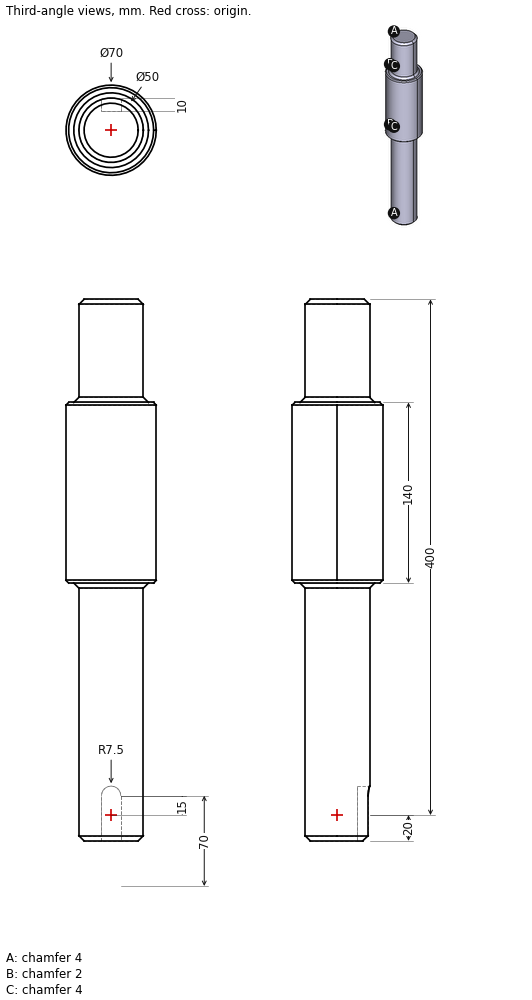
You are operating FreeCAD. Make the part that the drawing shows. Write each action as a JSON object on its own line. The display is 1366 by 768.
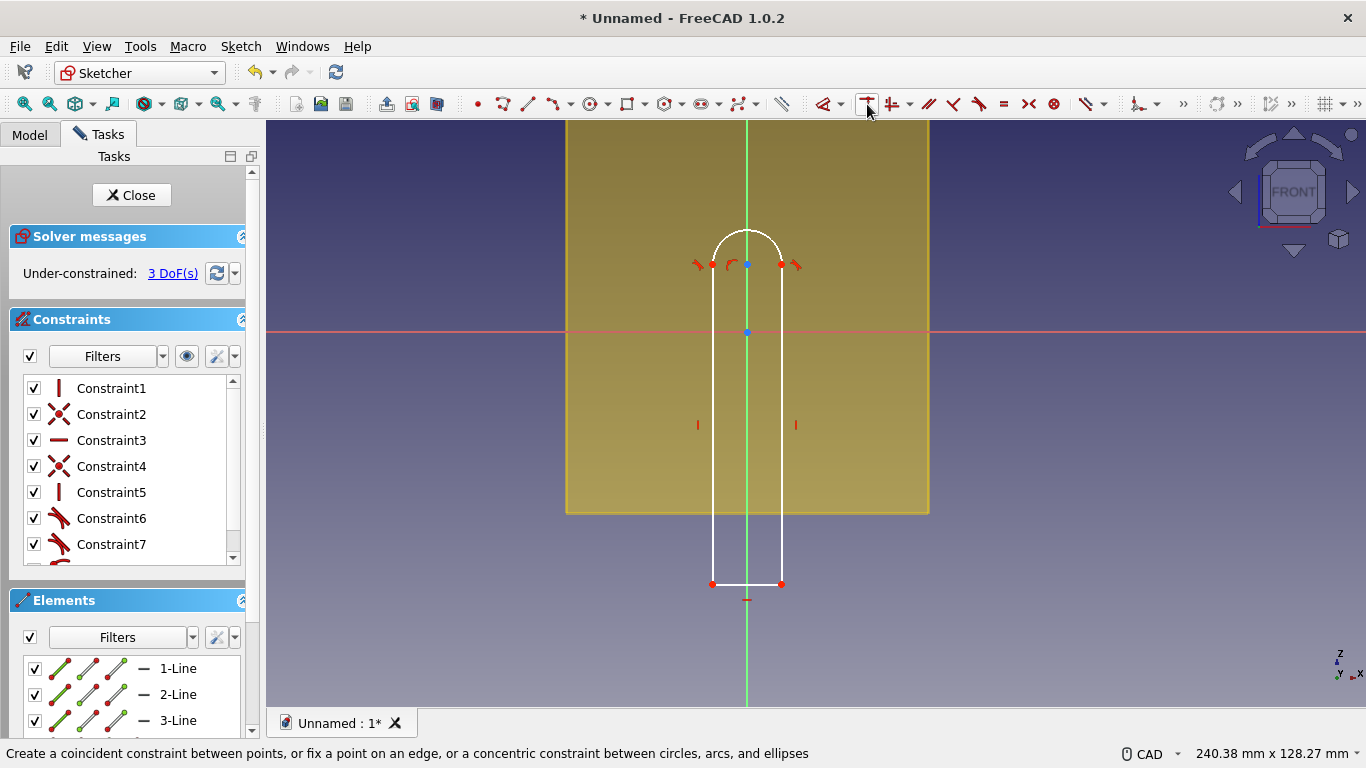
{"action": "left_click", "coordinate": [822, 104]}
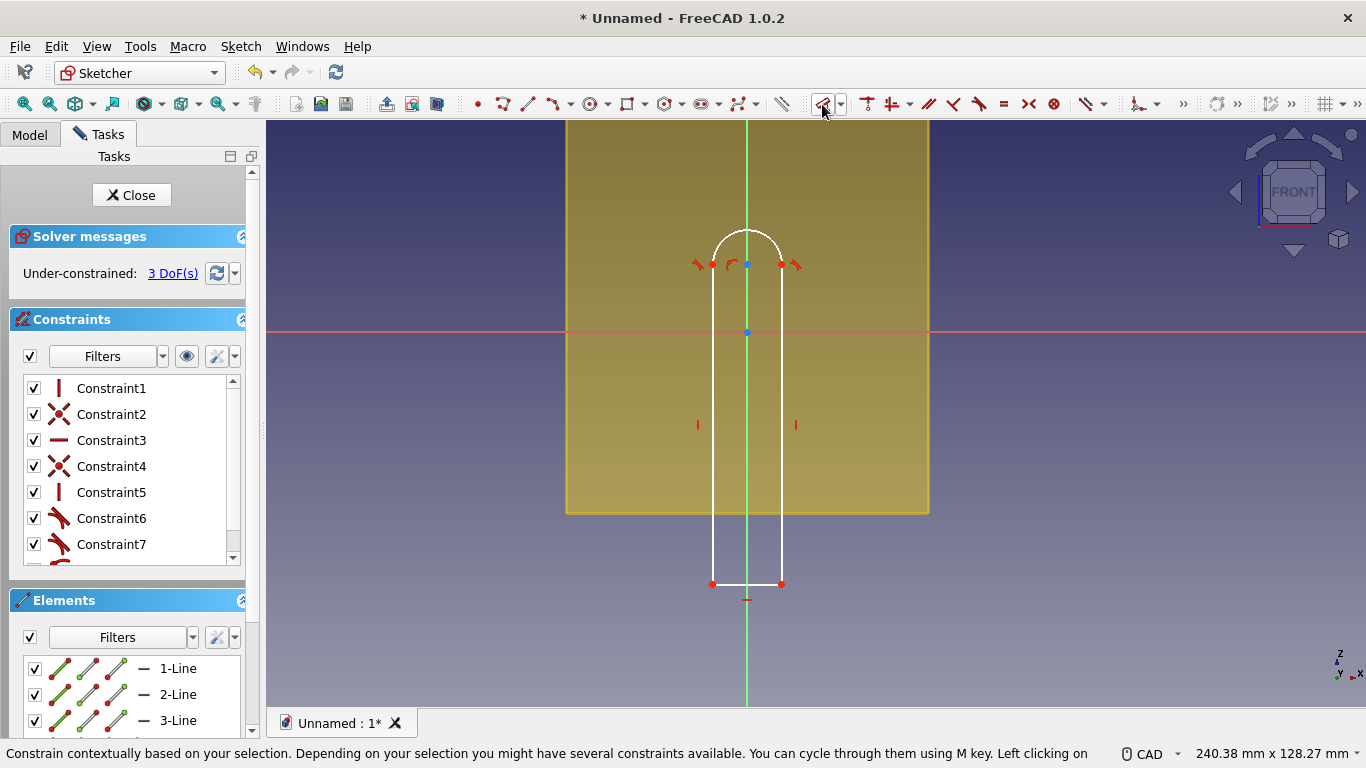
{"action": "left_click", "coordinate": [768, 237]}
{"action": "left_click", "coordinate": [787, 211]}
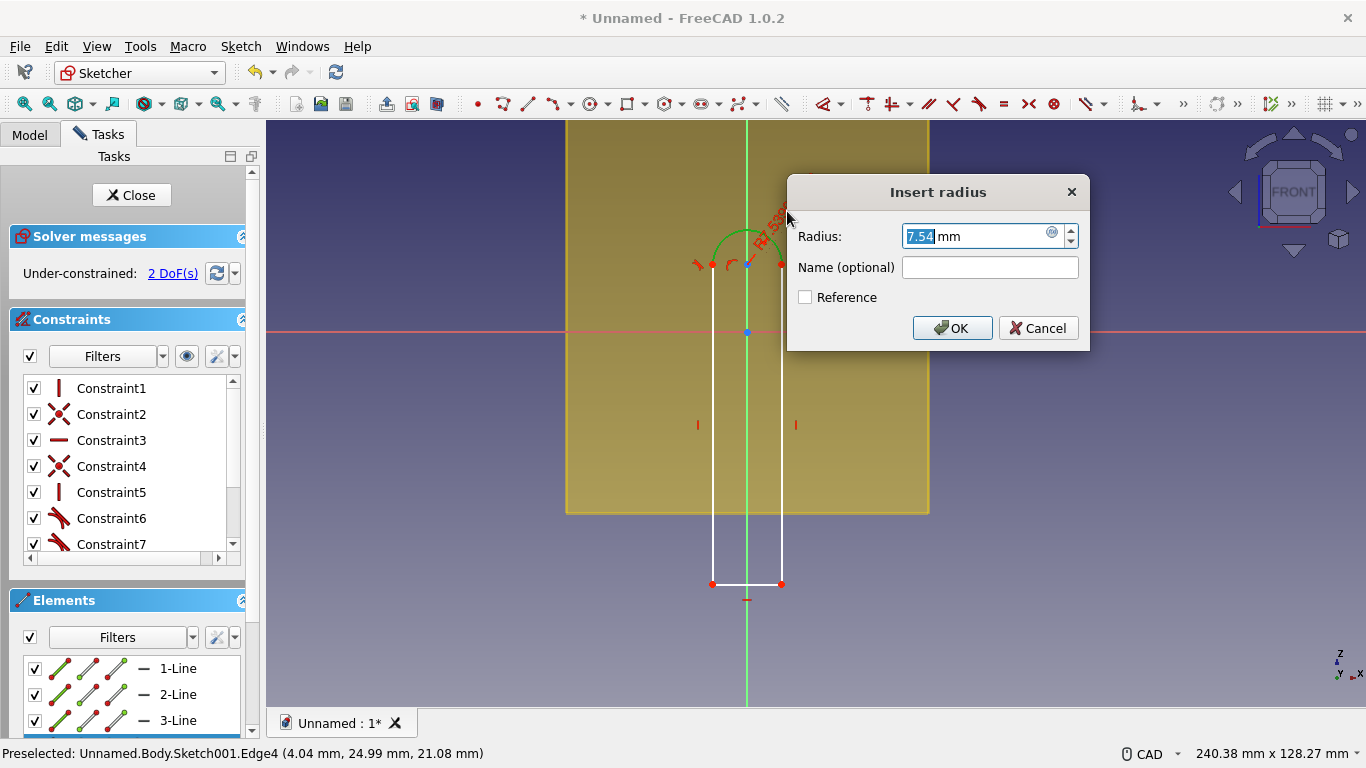
{"action": "type", "text": "7.5"}
{"action": "key", "text": "Return"}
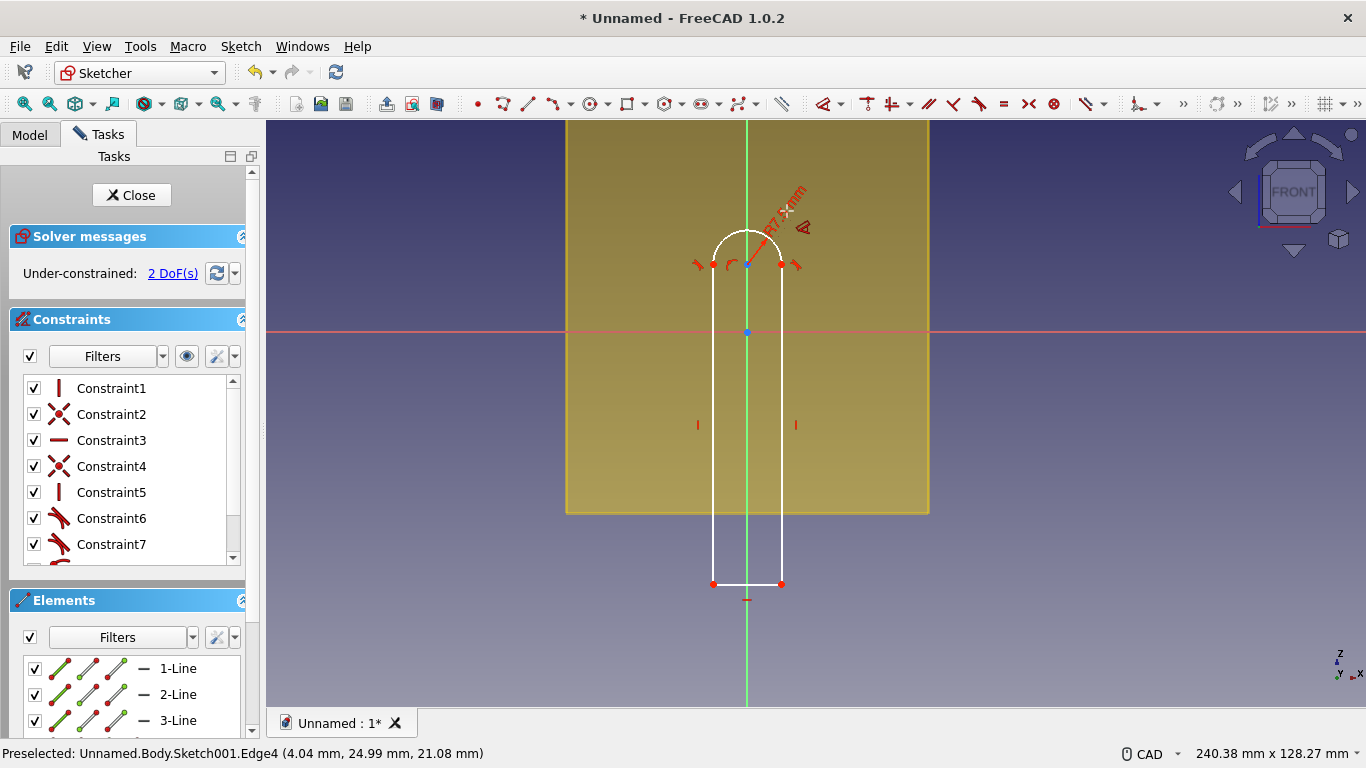
{"action": "left_click", "coordinate": [782, 361]}
{"action": "left_click", "coordinate": [816, 425]}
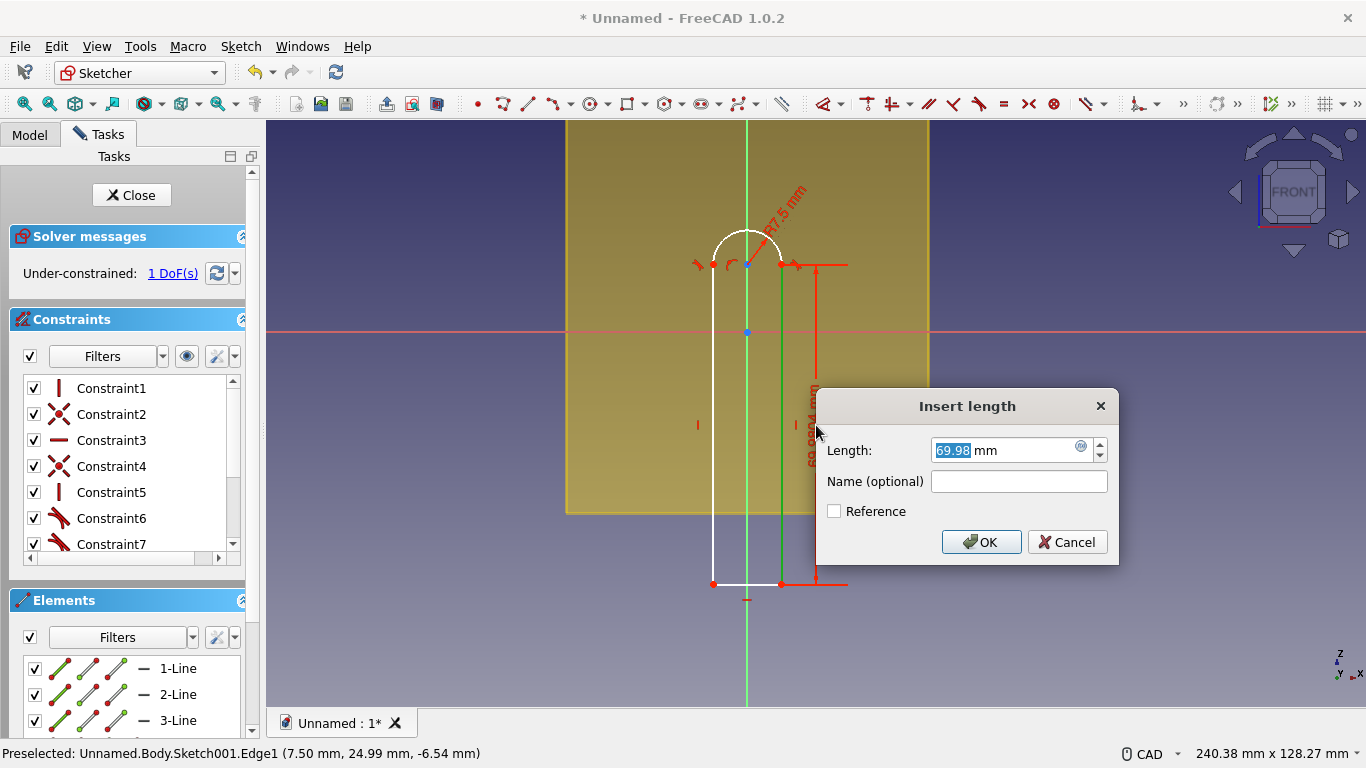
{"action": "type", "text": "70"}
{"action": "key", "text": "Return"}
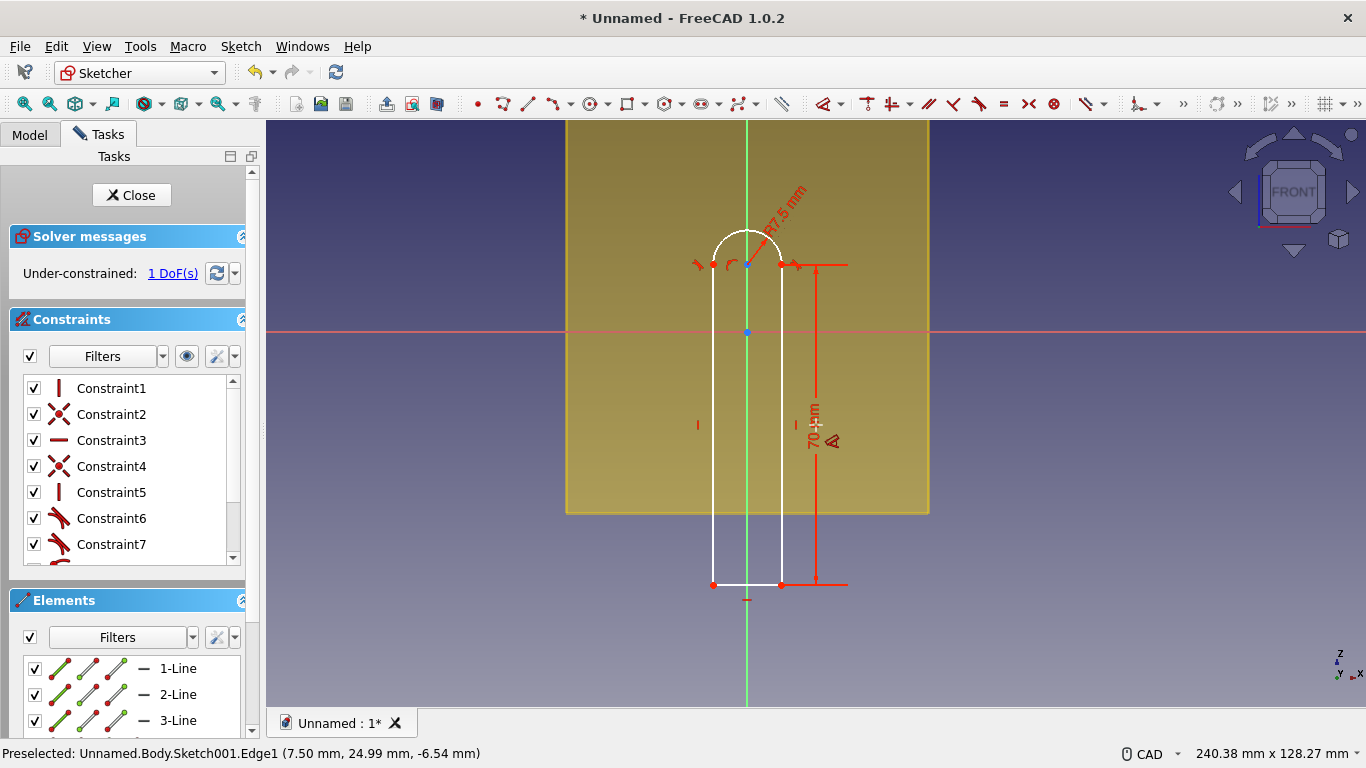
{"action": "left_click", "coordinate": [782, 265]}
{"action": "left_click", "coordinate": [816, 298]}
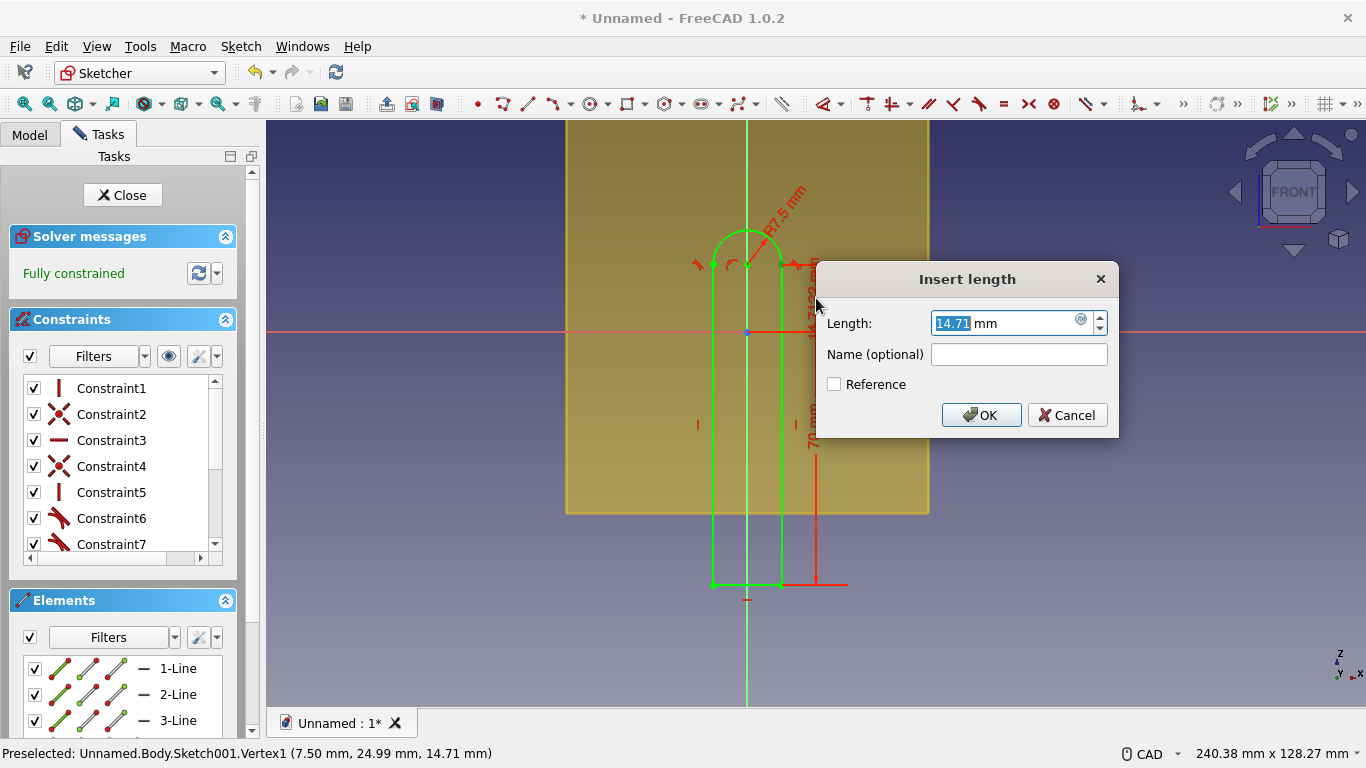
{"action": "type", "text": "15"}
{"action": "key", "text": "Return"}
{"action": "key", "text": "Escape"}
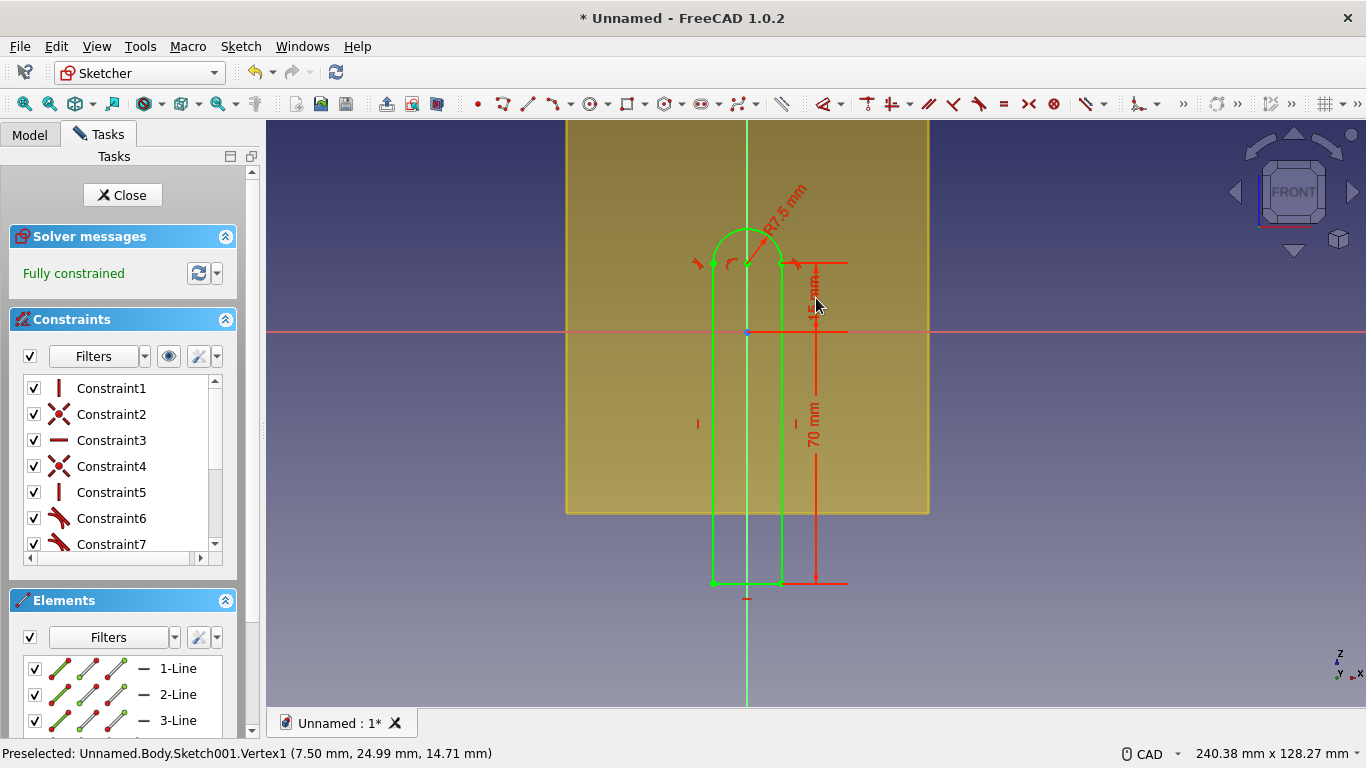
{"action": "left_click", "coordinate": [123, 195]}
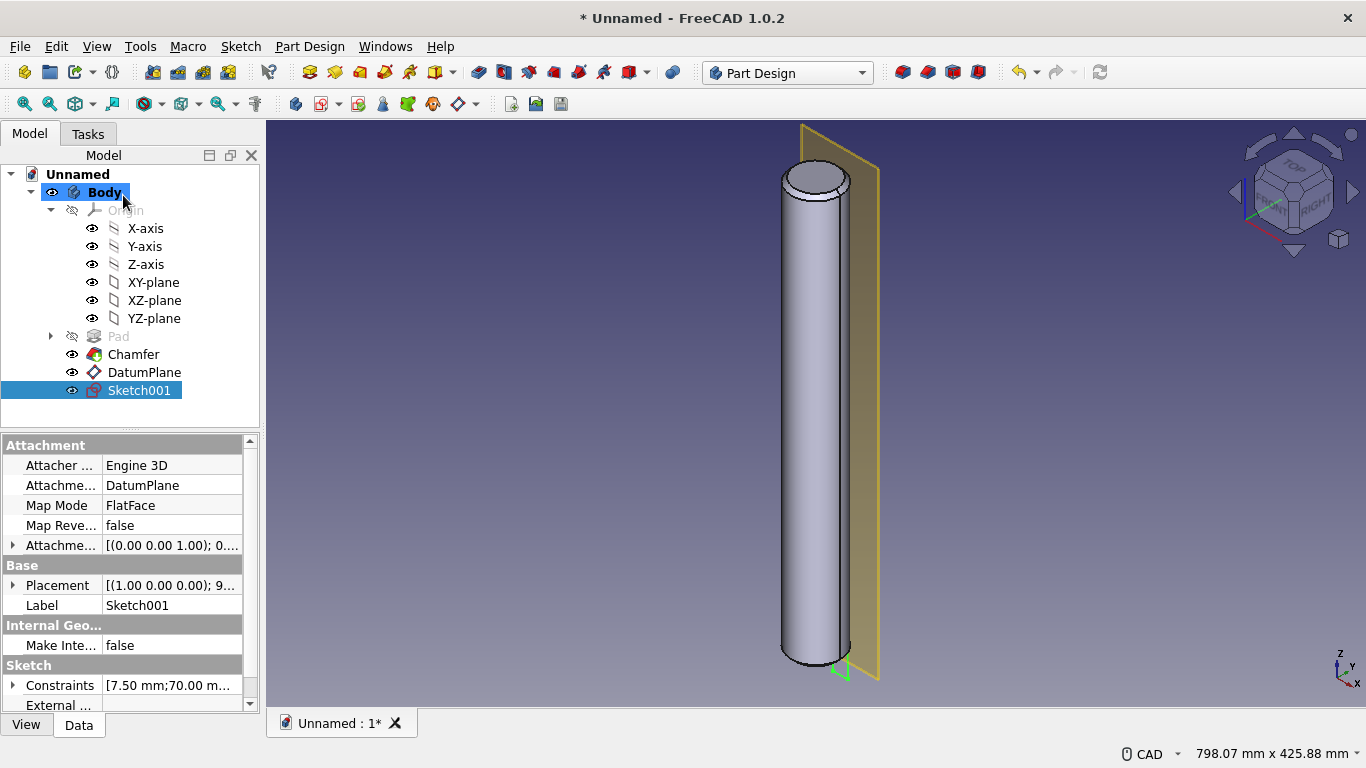
{"action": "left_click", "coordinate": [479, 72]}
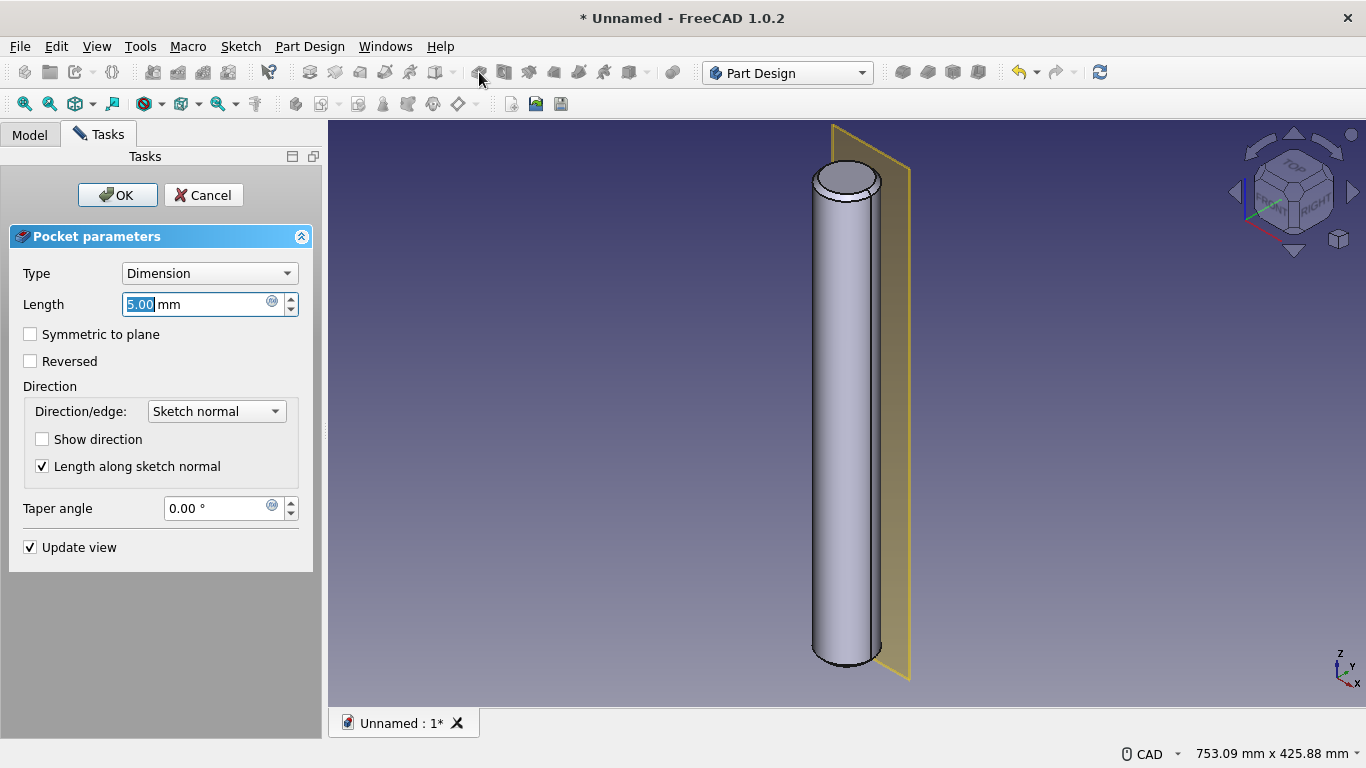
{"action": "type", "text": "10"}
{"action": "key", "text": "Tab"}